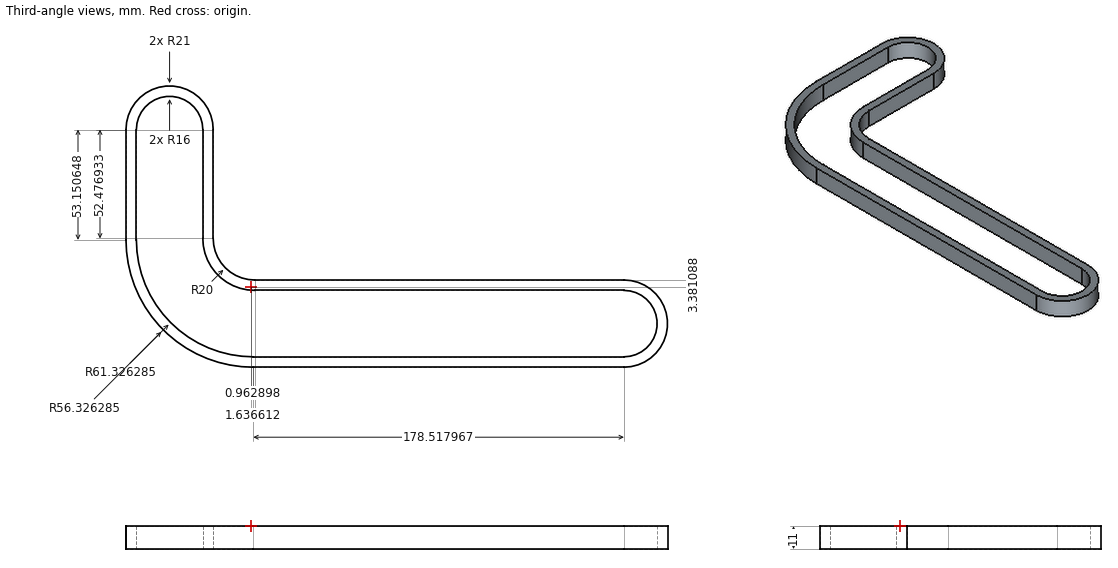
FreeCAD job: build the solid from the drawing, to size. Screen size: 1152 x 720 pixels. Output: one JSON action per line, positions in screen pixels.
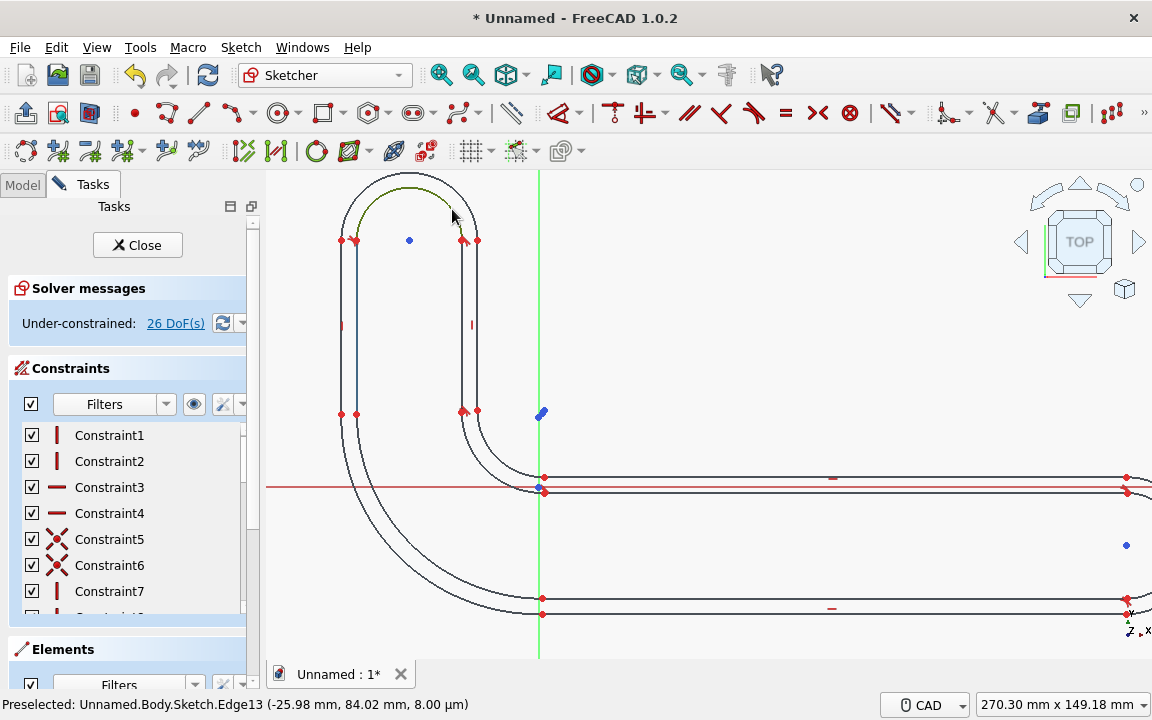
{"action": "left_click", "coordinate": [754, 114]}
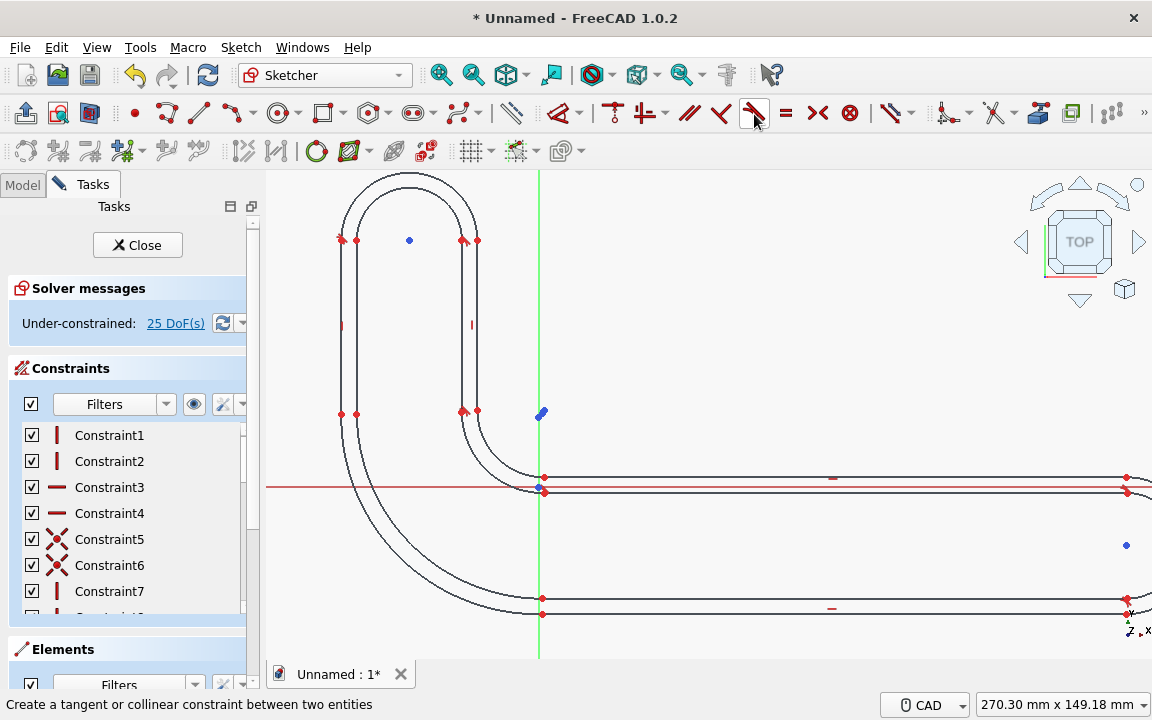
{"action": "left_click", "coordinate": [462, 292]}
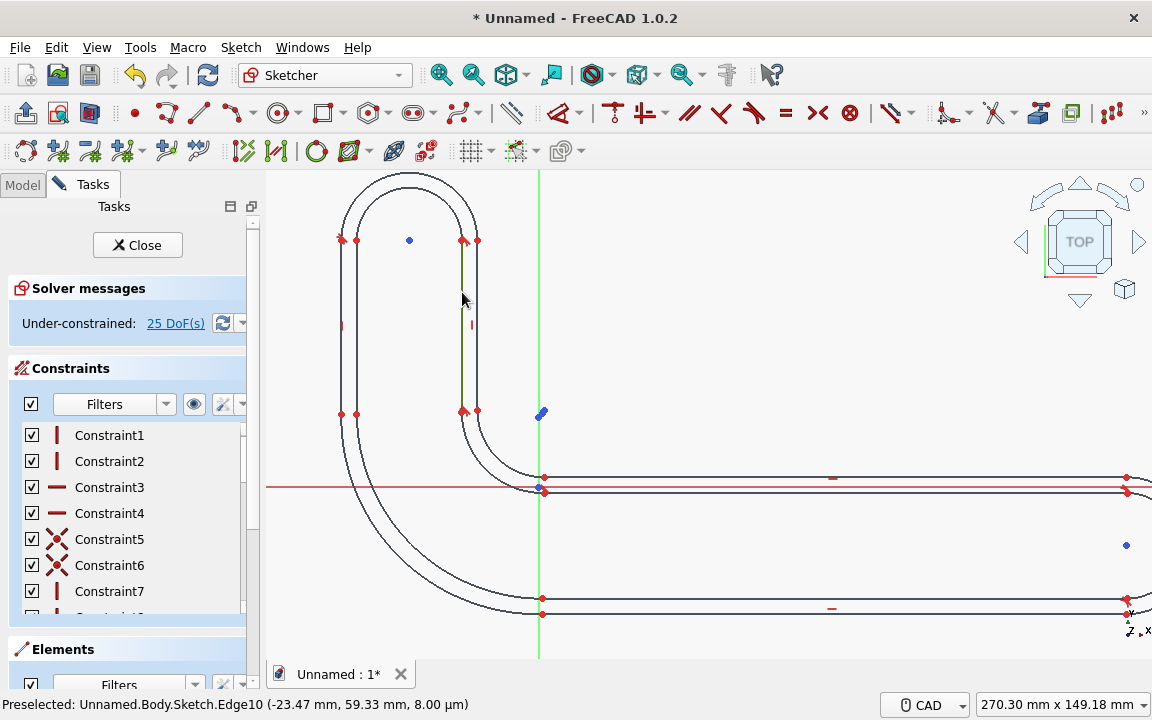
{"action": "left_click", "coordinate": [452, 209]}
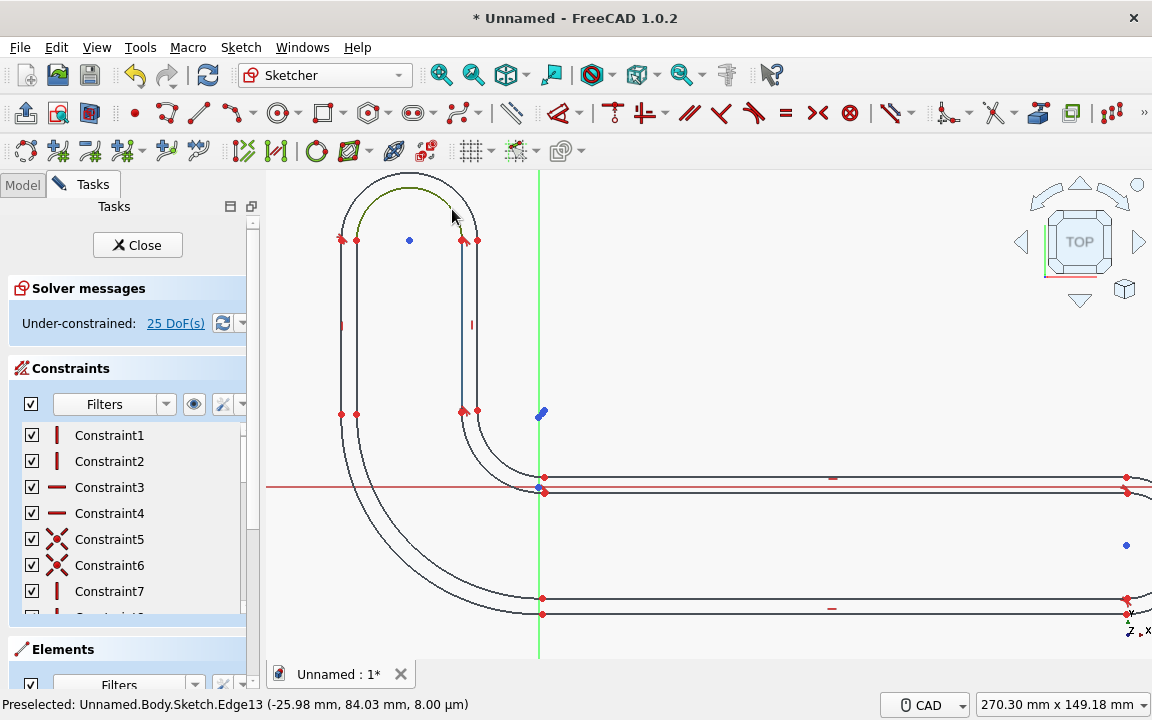
{"action": "left_click", "coordinate": [754, 114]}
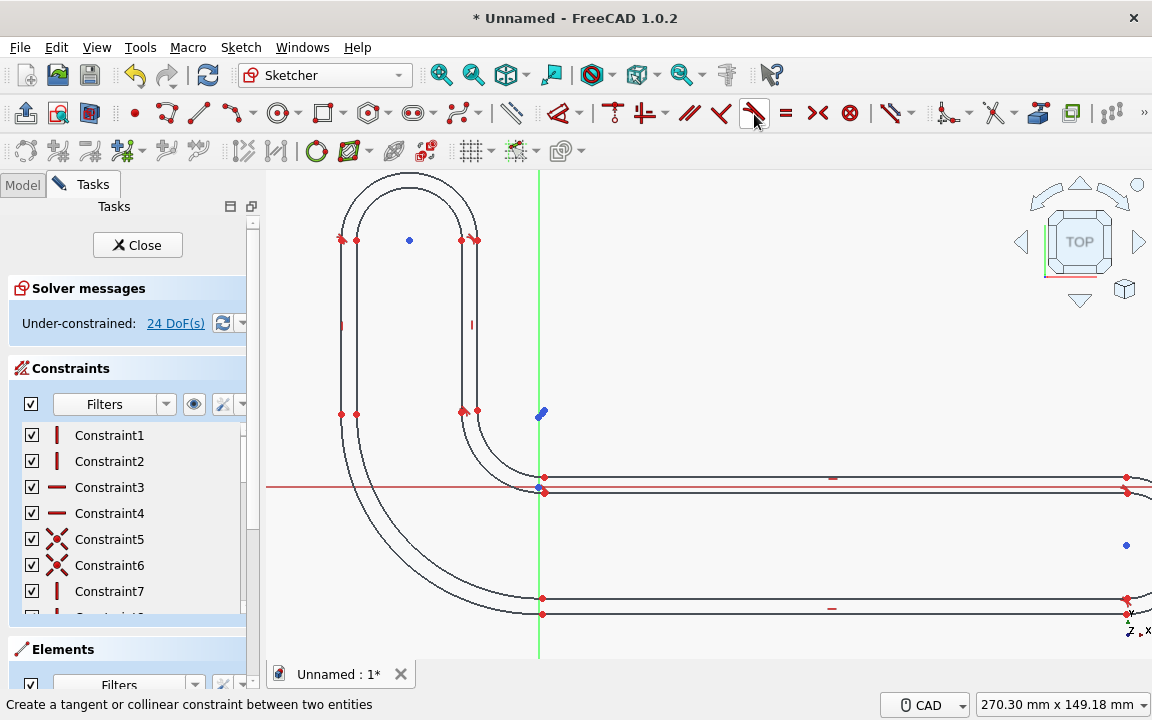
{"action": "left_click", "coordinate": [462, 292]}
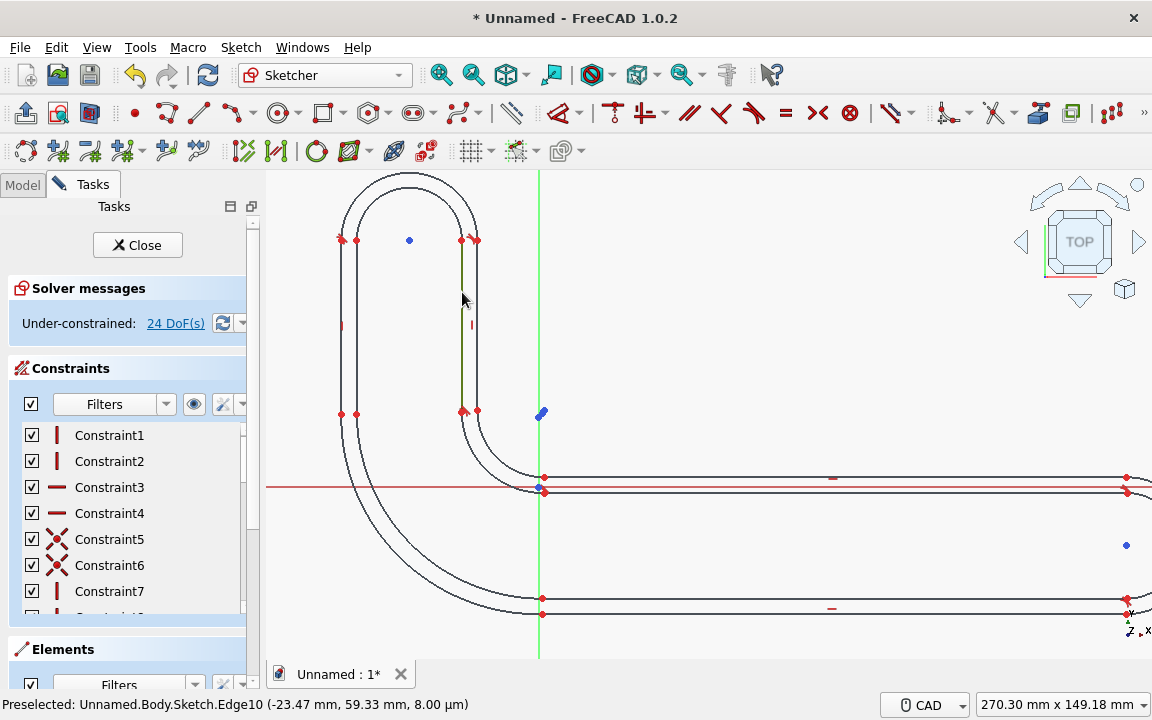
{"action": "left_click", "coordinate": [471, 449]}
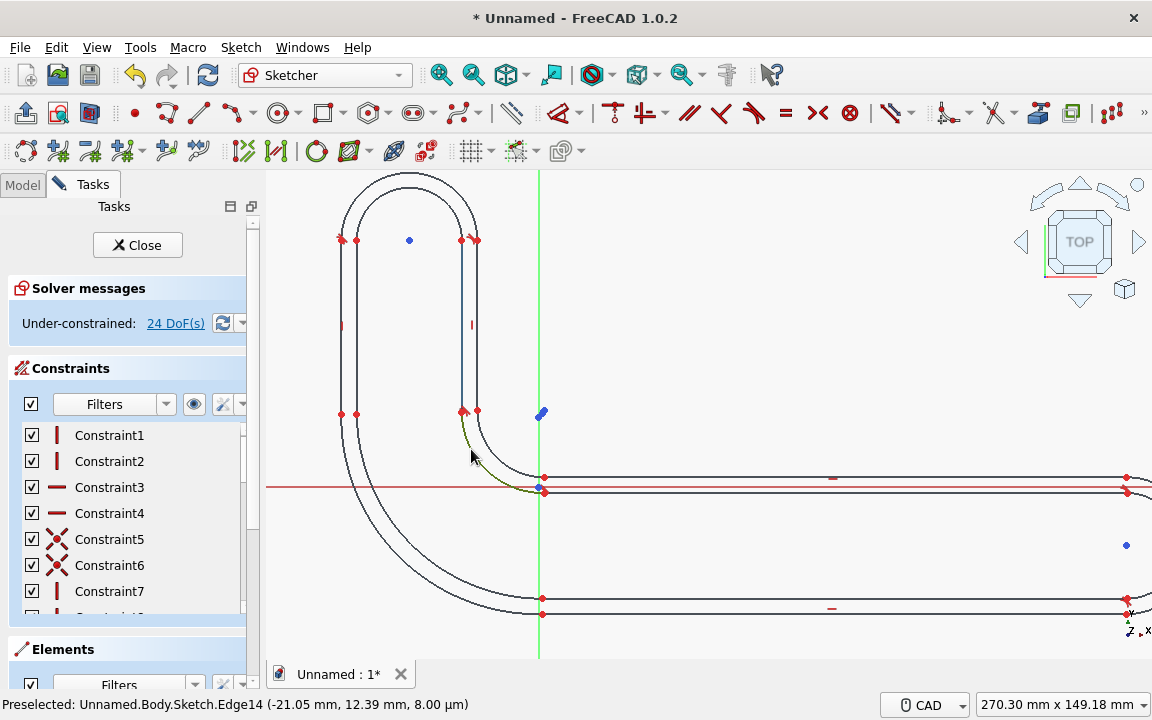
{"action": "left_click", "coordinate": [754, 114]}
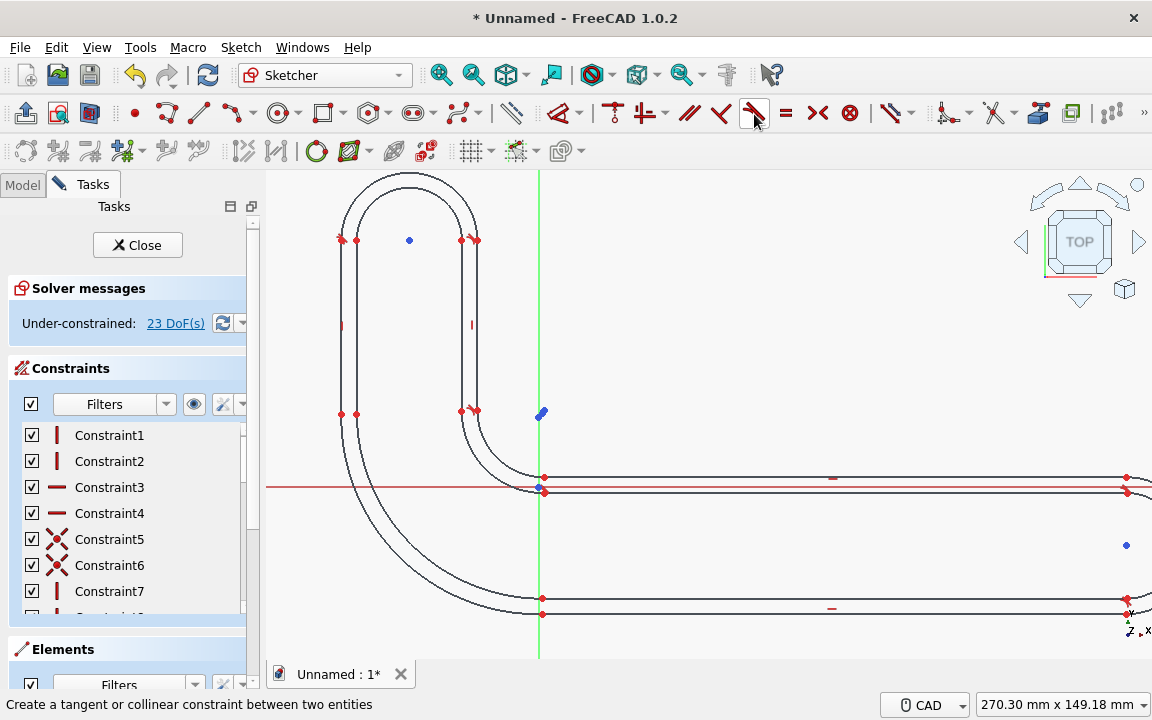
{"action": "scroll", "coordinate": [719, 493], "scroll_direction": "up", "scroll_amount": 5}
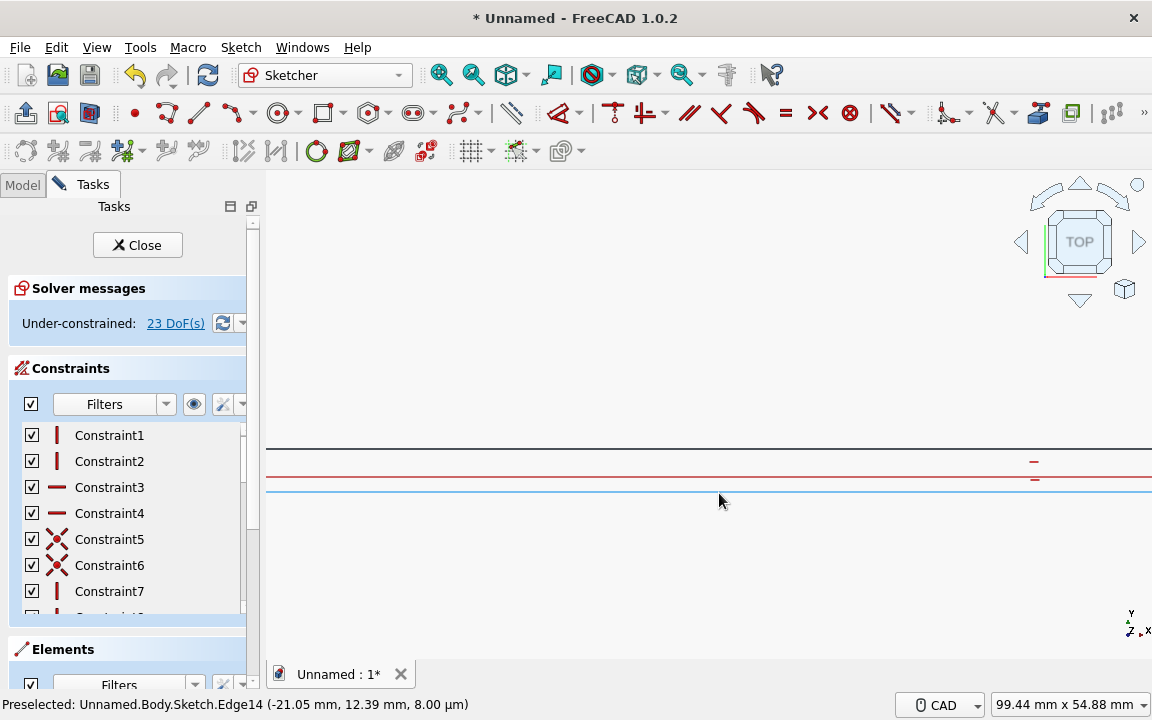
{"action": "left_click", "coordinate": [718, 492]}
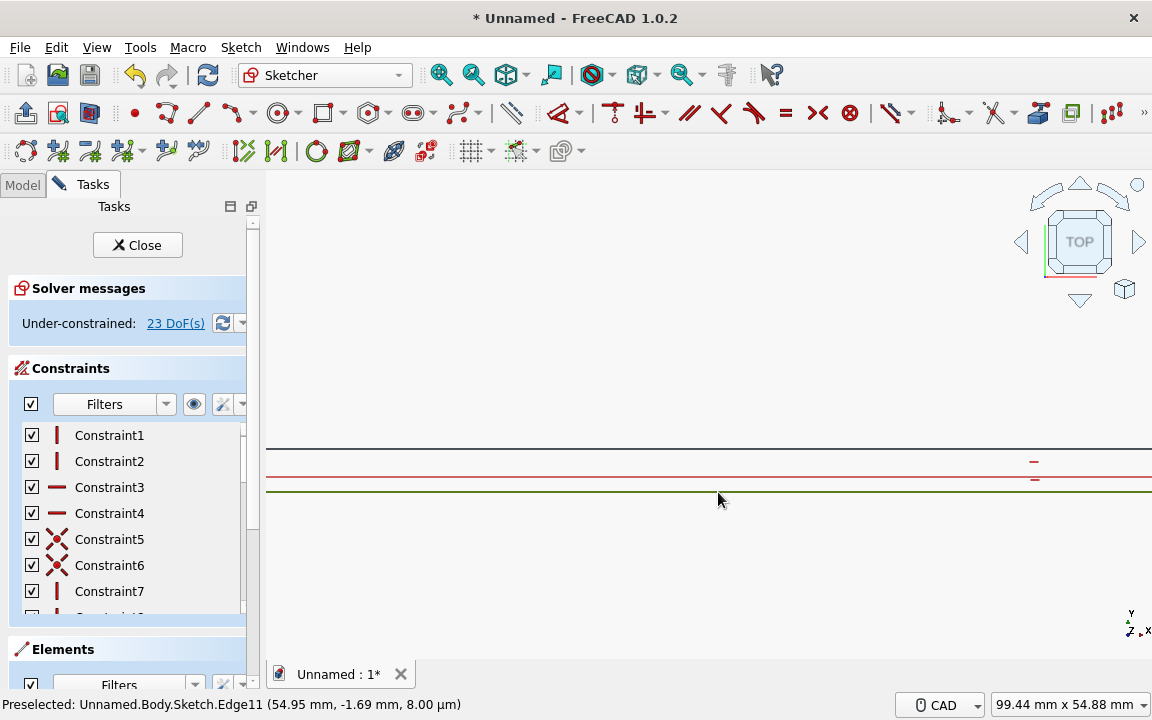
{"action": "scroll", "coordinate": [587, 464], "scroll_direction": "down", "scroll_amount": 8}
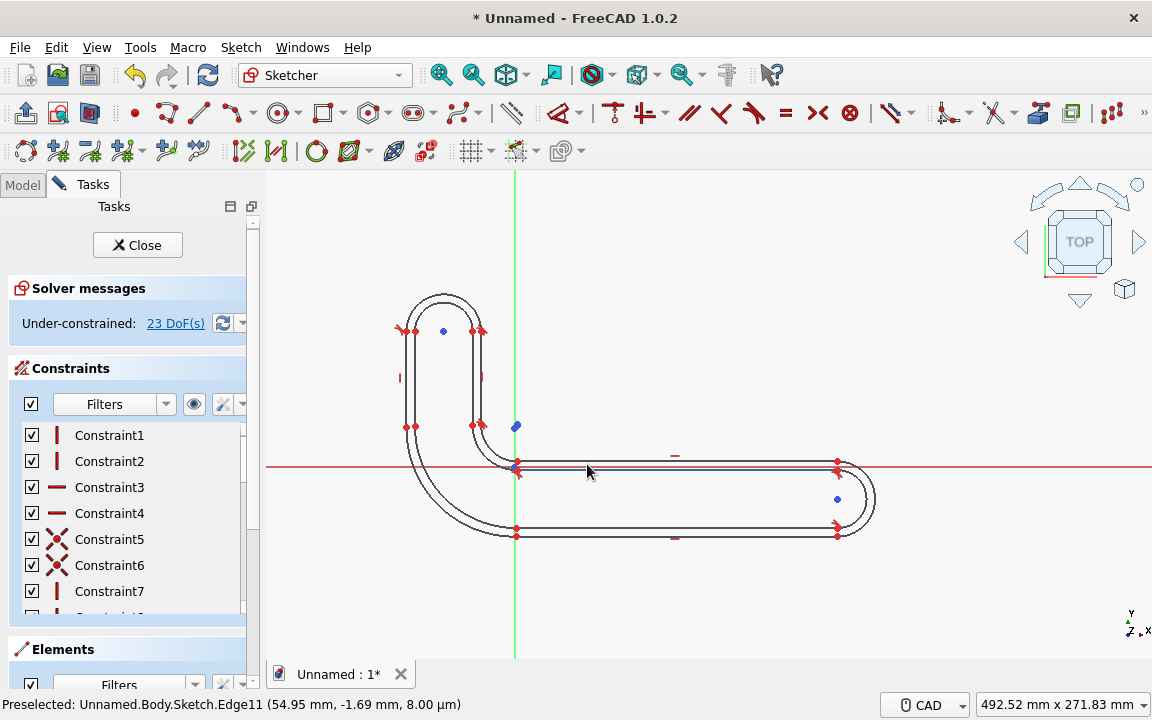
{"action": "scroll", "coordinate": [478, 446], "scroll_direction": "up", "scroll_amount": 3}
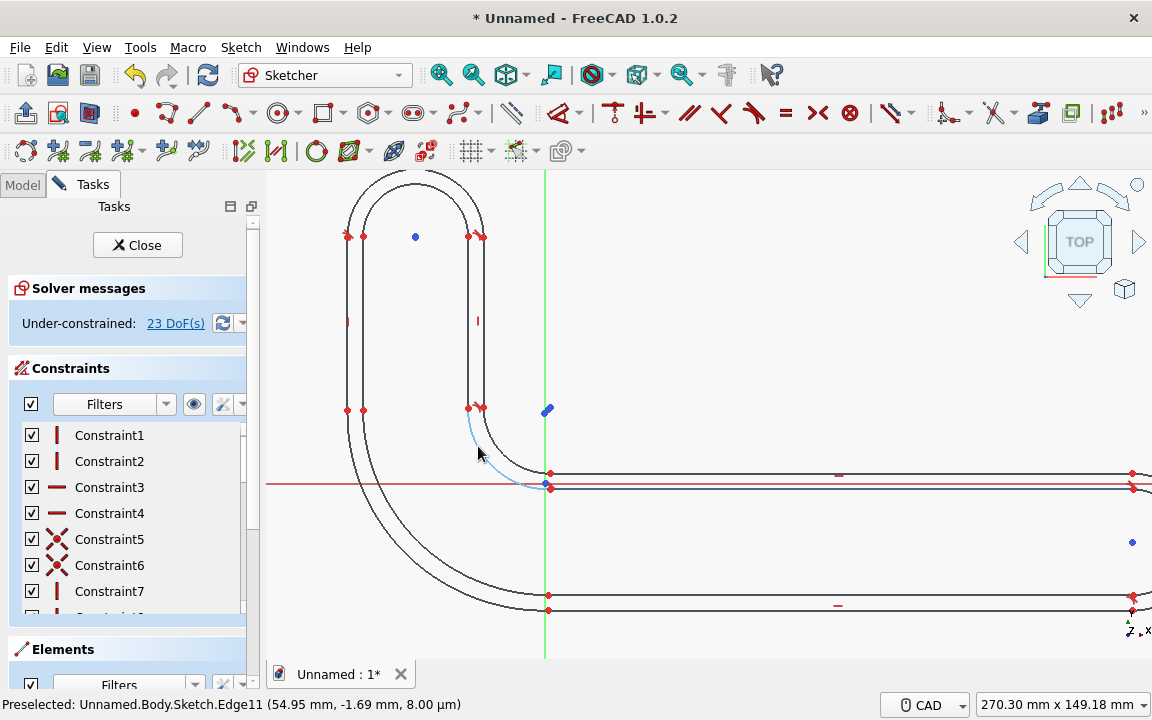
{"action": "left_click", "coordinate": [477, 445]}